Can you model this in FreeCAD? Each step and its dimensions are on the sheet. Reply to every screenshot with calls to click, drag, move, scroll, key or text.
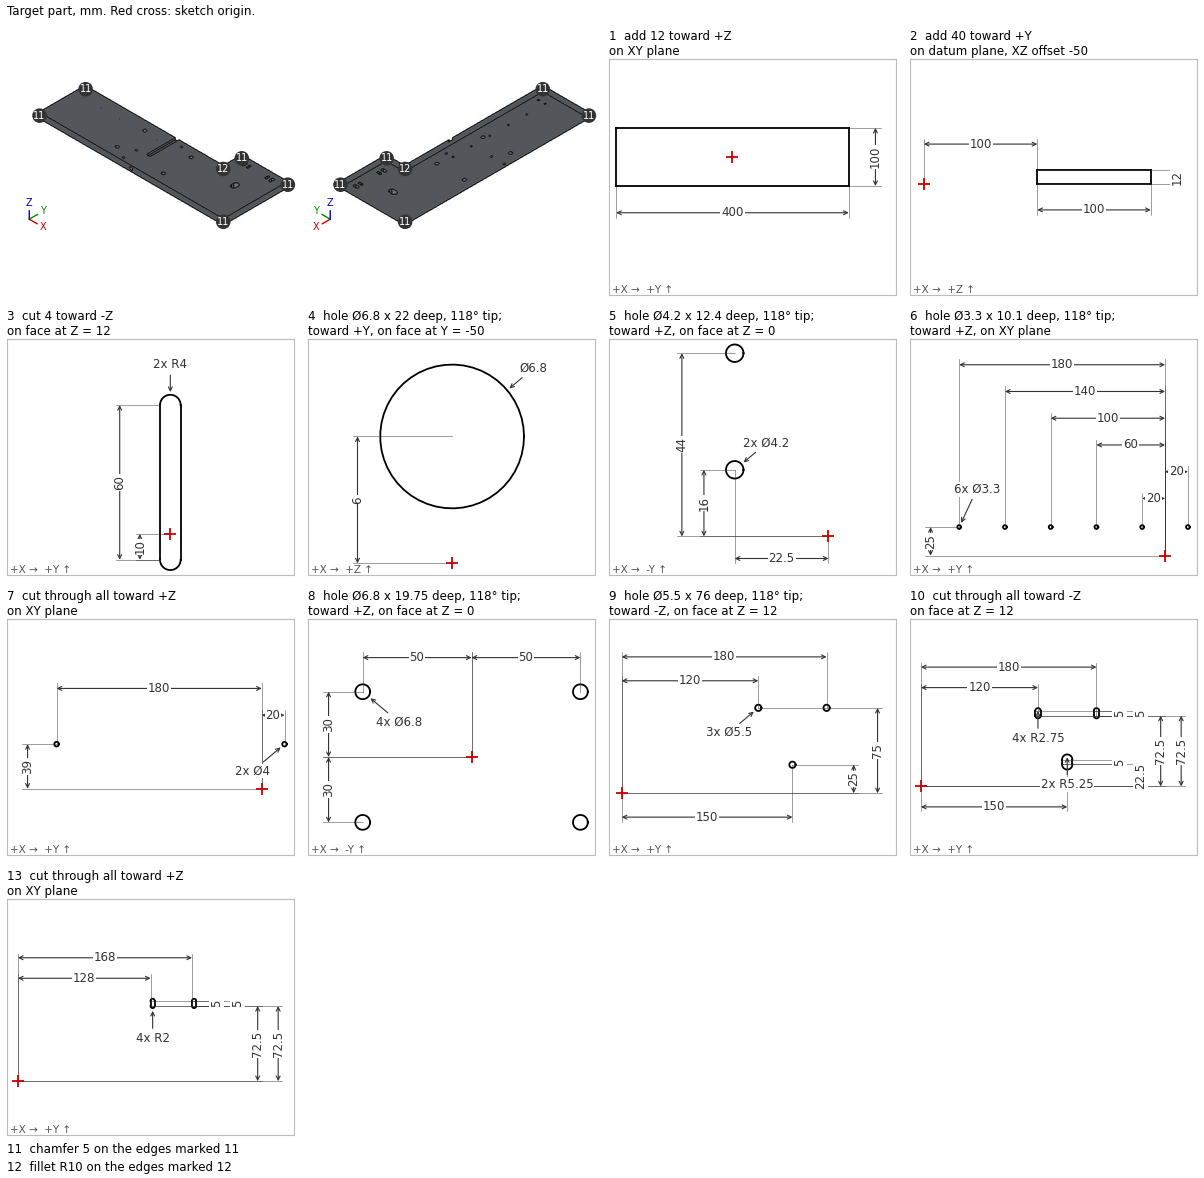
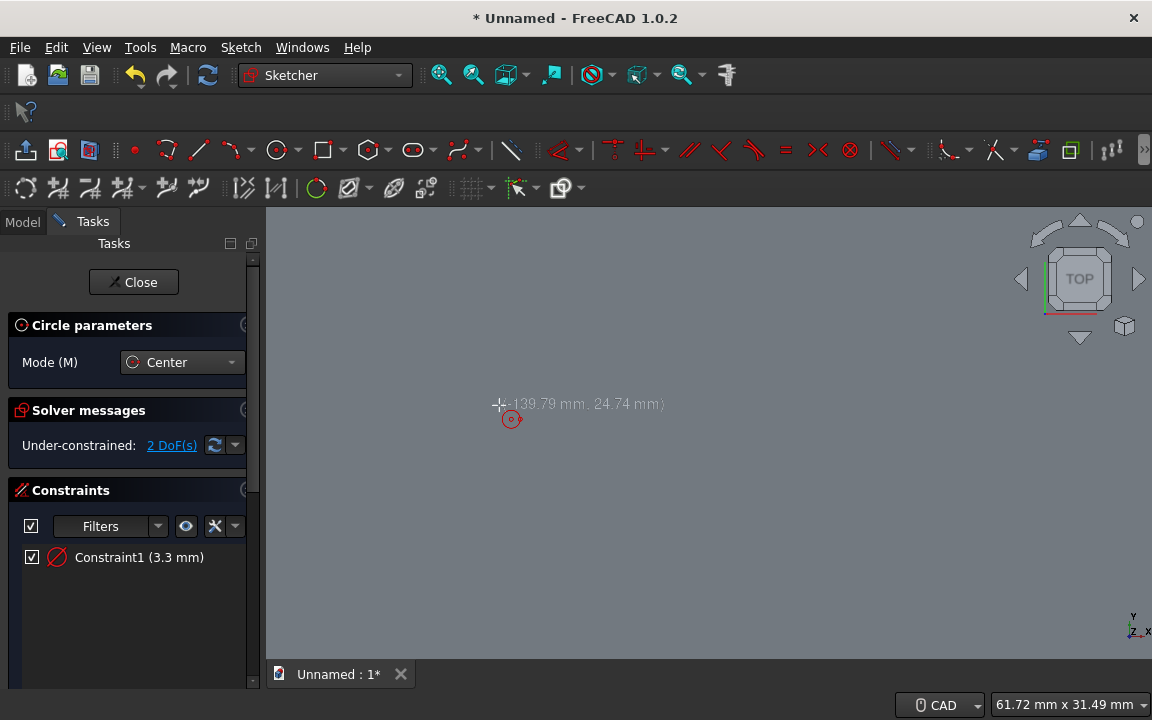
scroll(499, 405, down, 9)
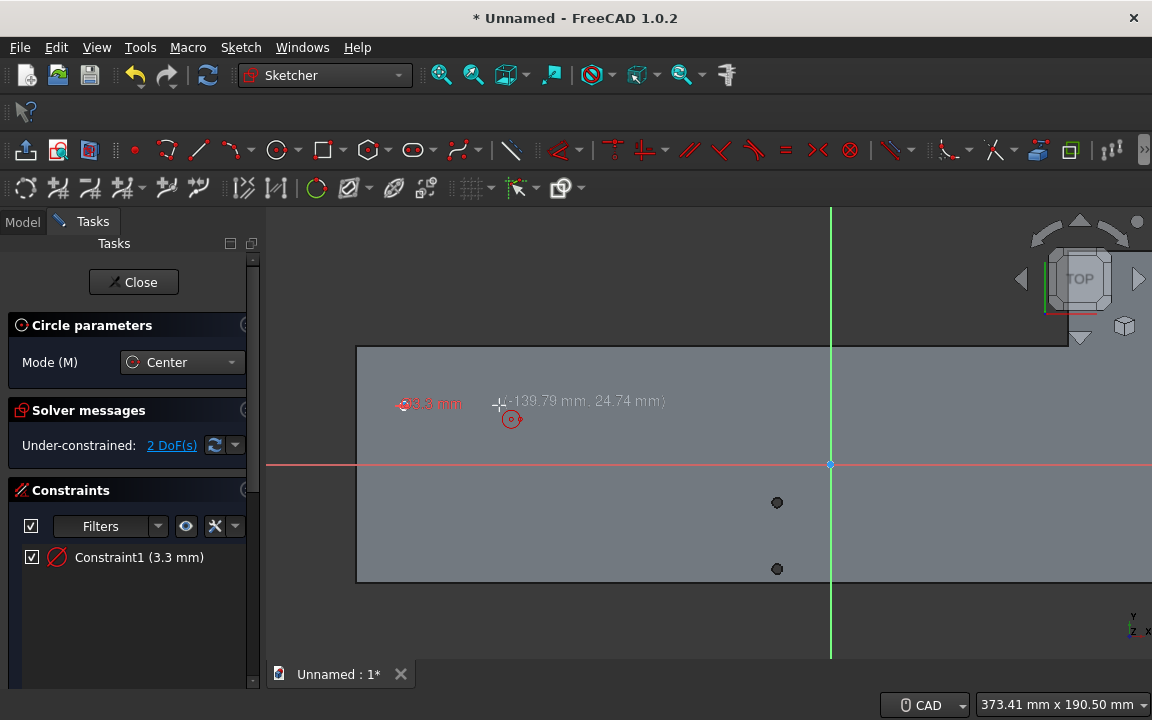
click(499, 405)
move(501, 403)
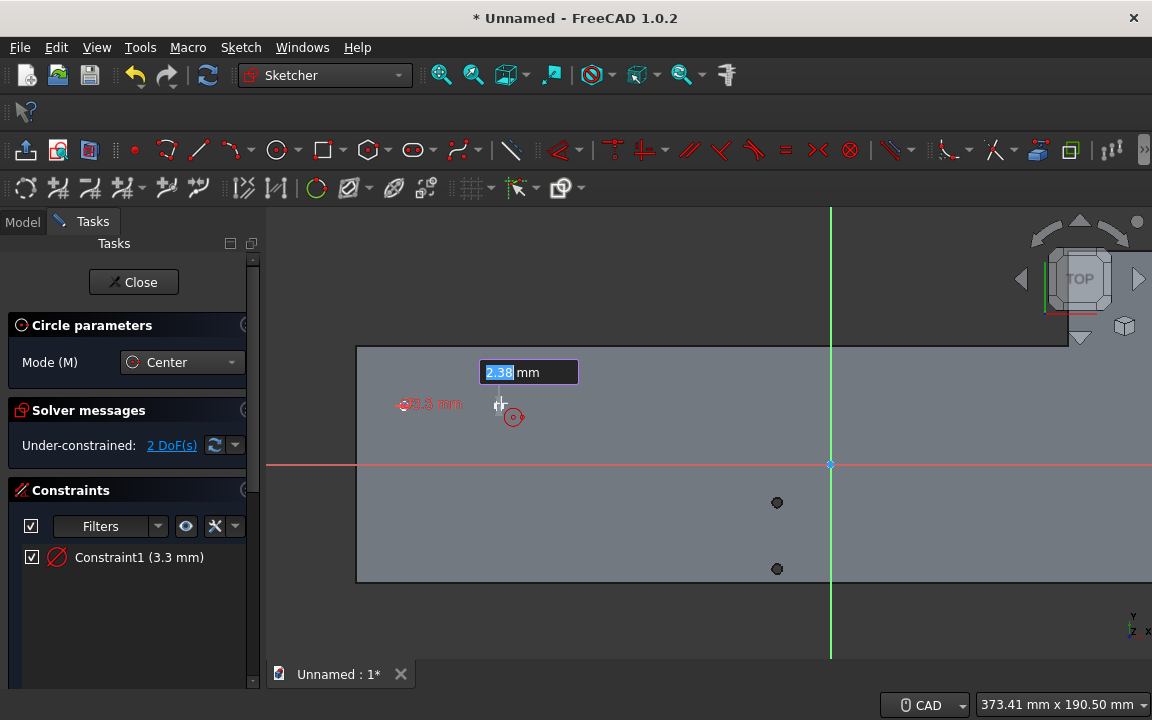
text(3.3)
key(Return)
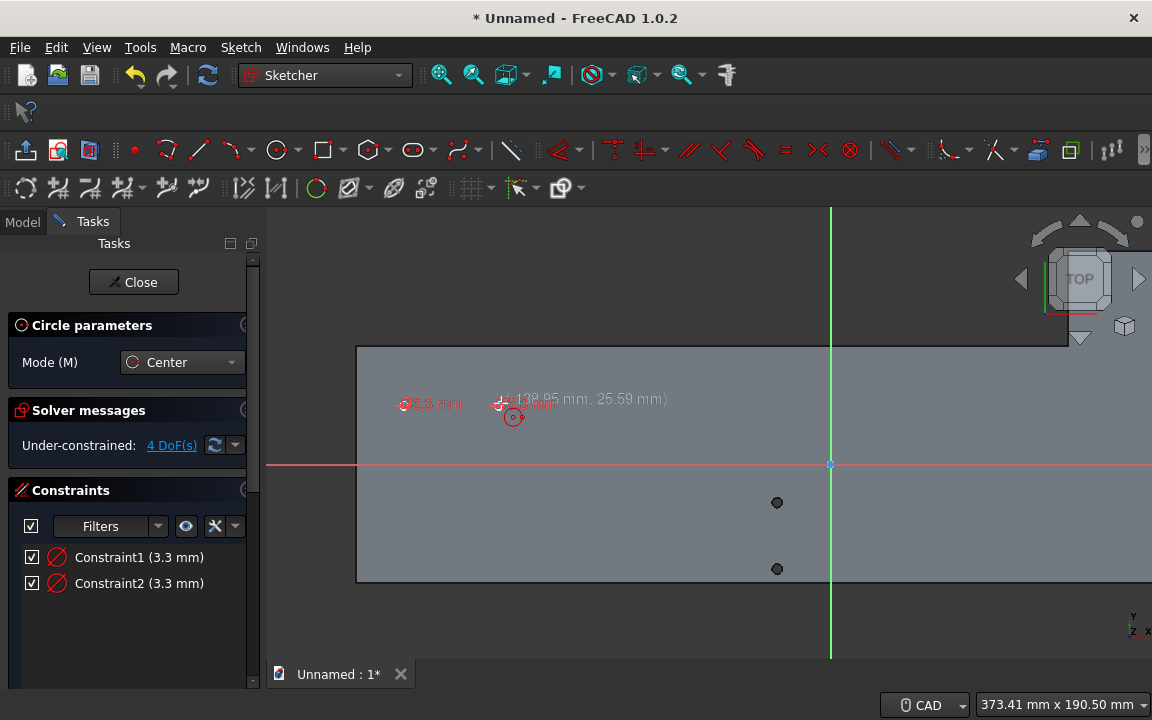
scroll(593, 405, up, 9)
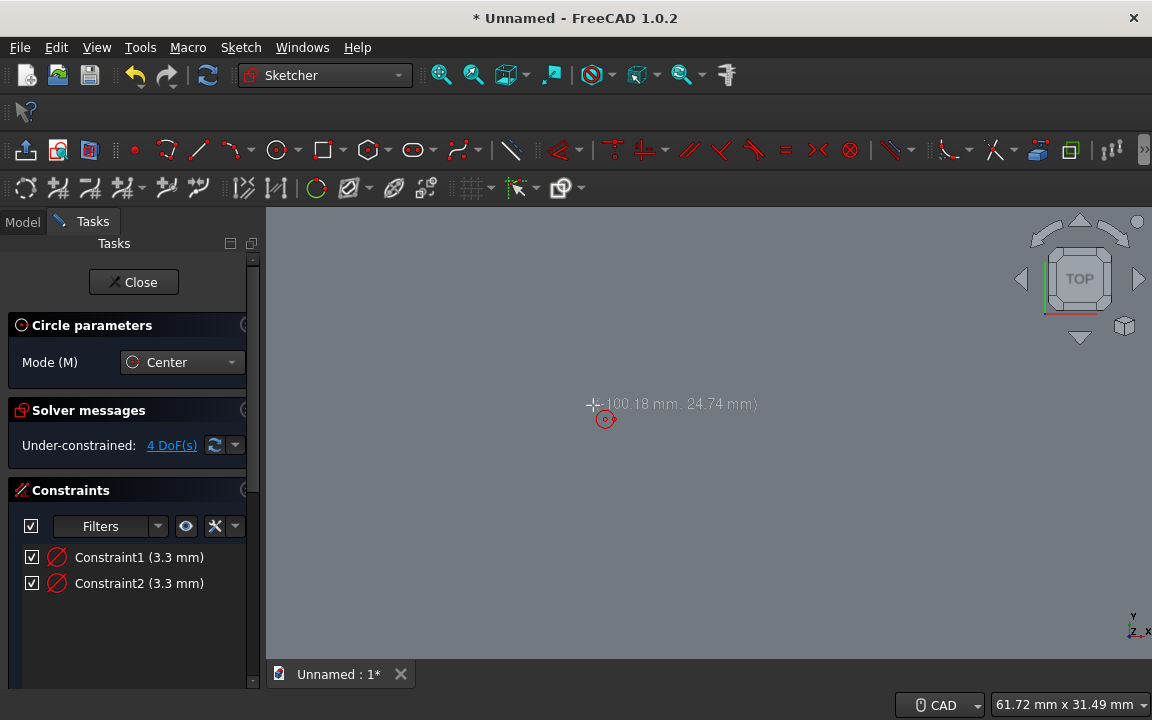
scroll(593, 405, down, 9)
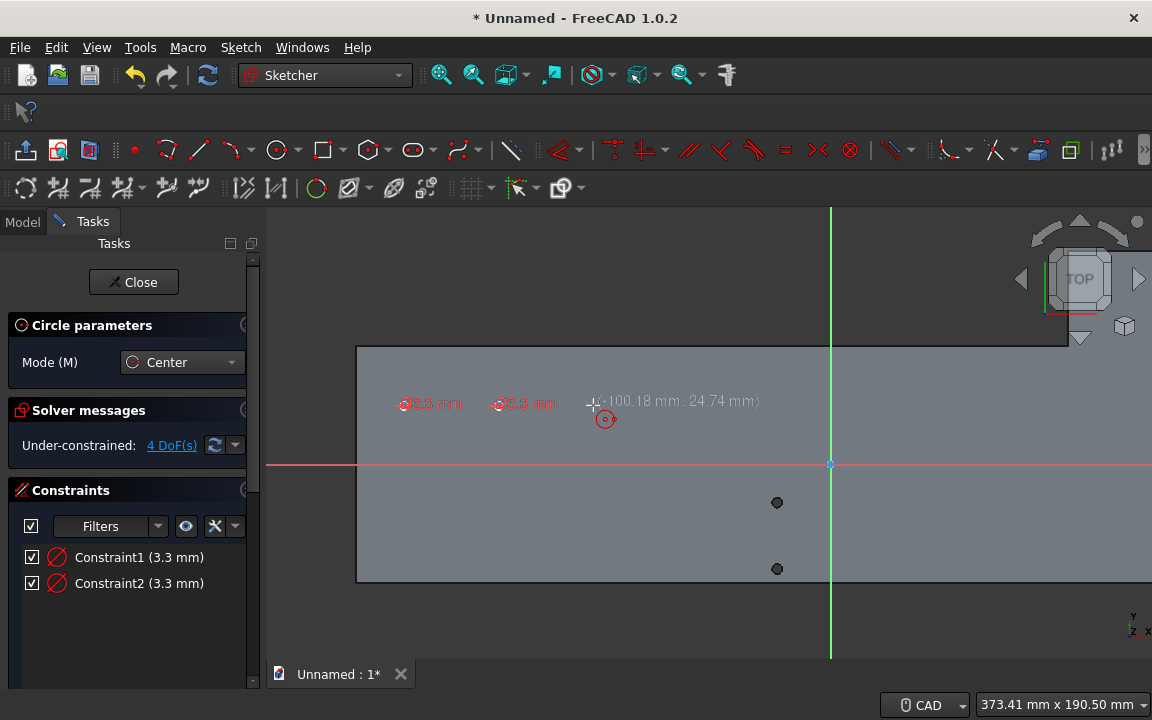
click(593, 405)
move(596, 403)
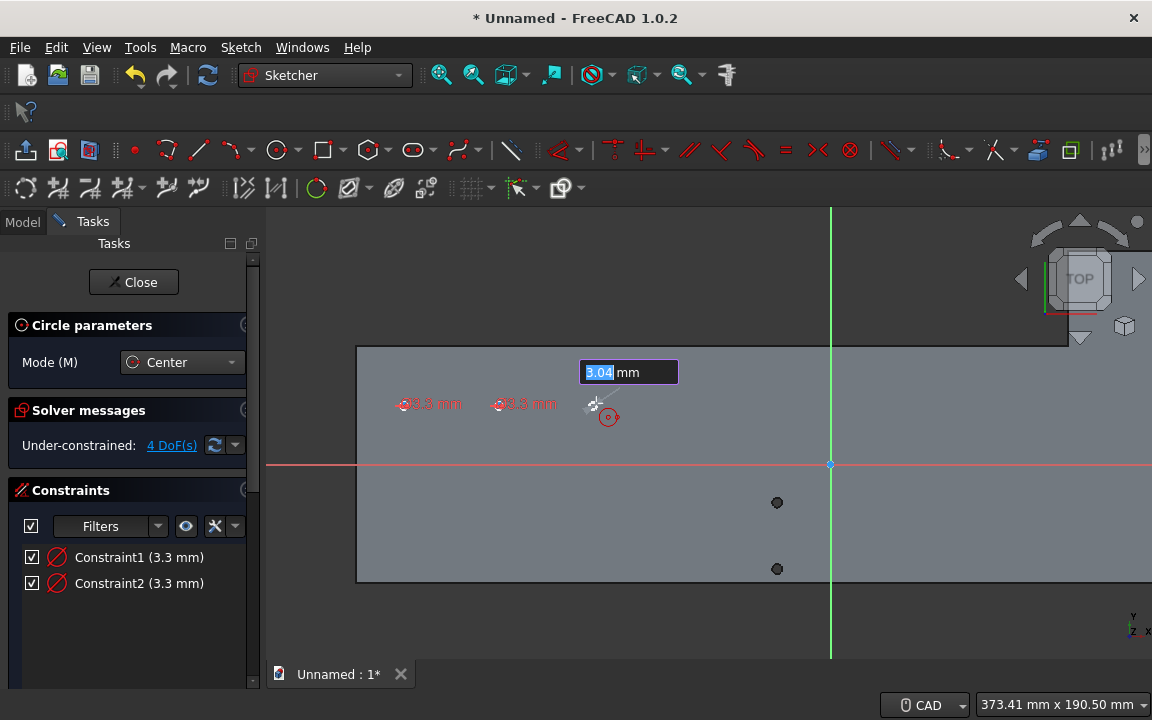
text(3.3)
key(Return)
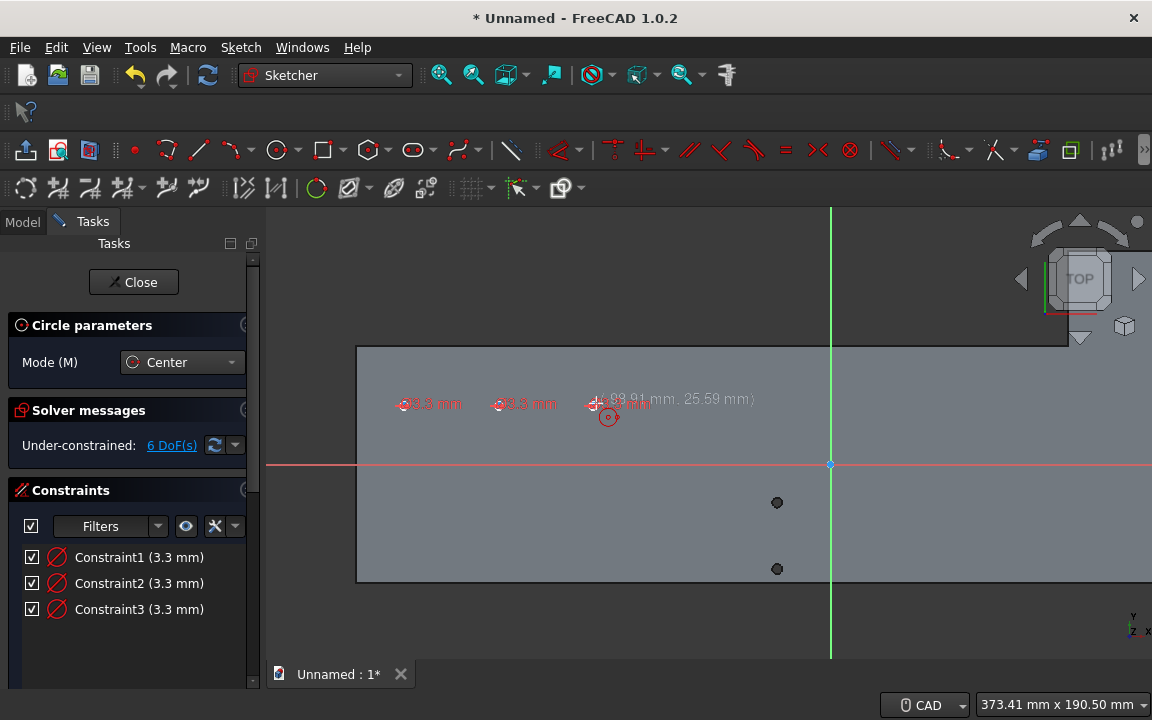
scroll(688, 405, up, 9)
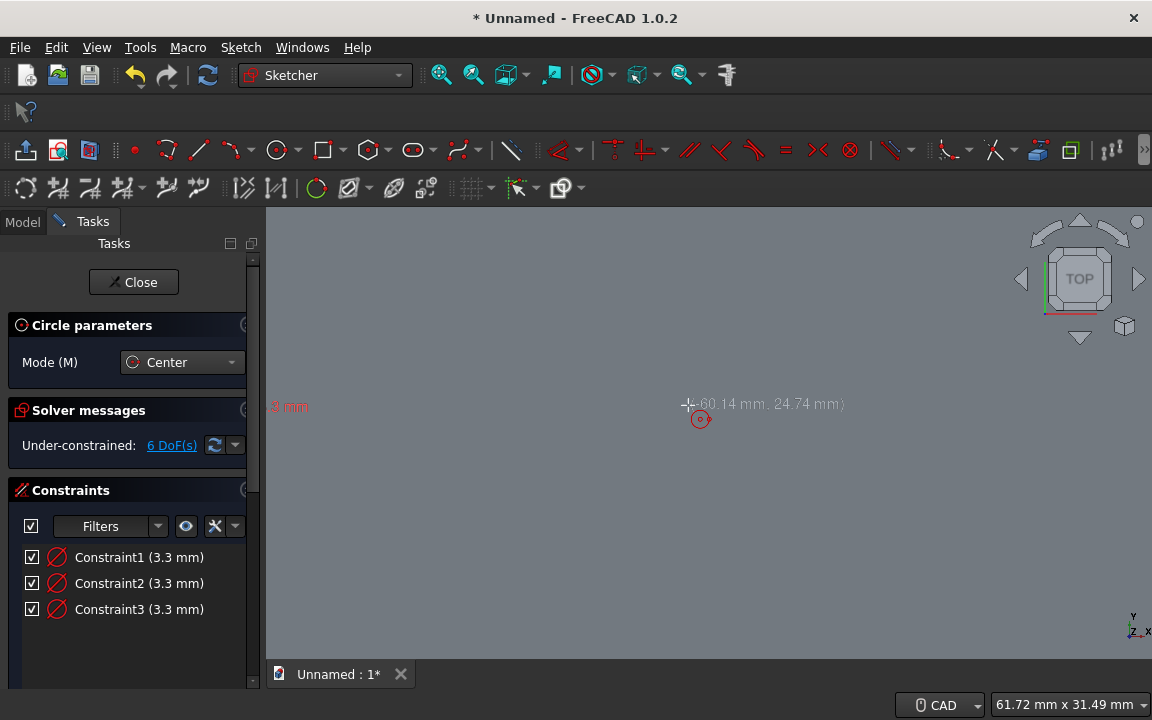
scroll(688, 405, down, 9)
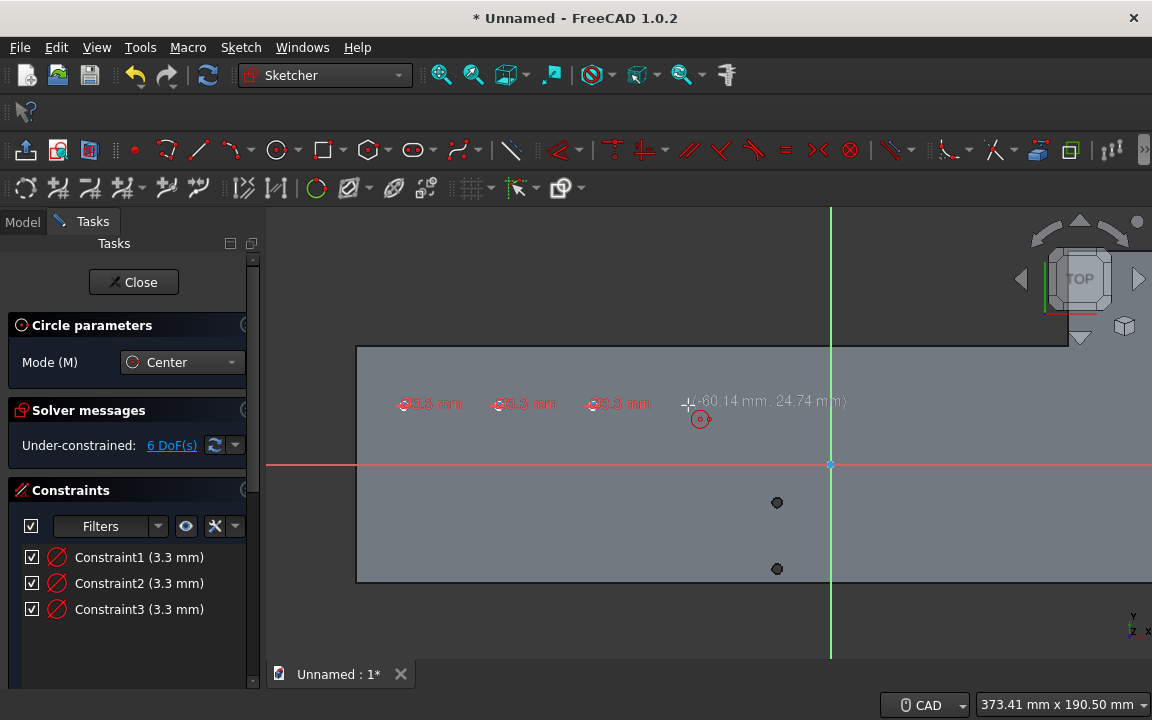
click(688, 405)
move(691, 403)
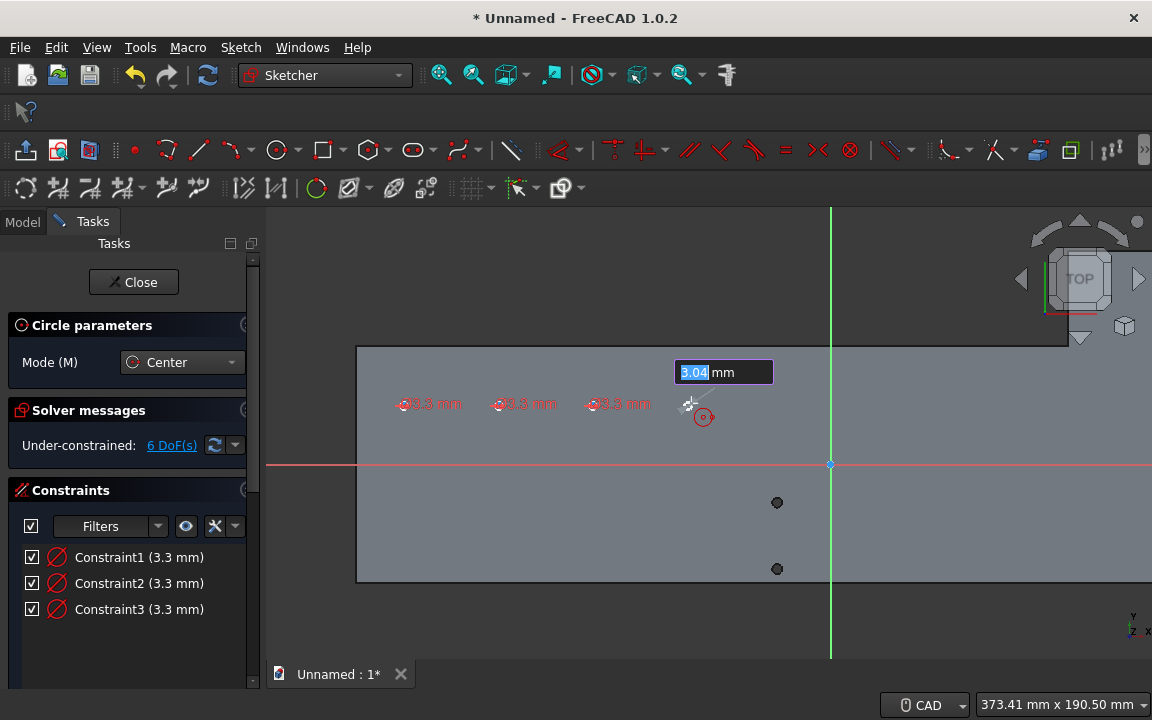
text(3.3)
key(Return)